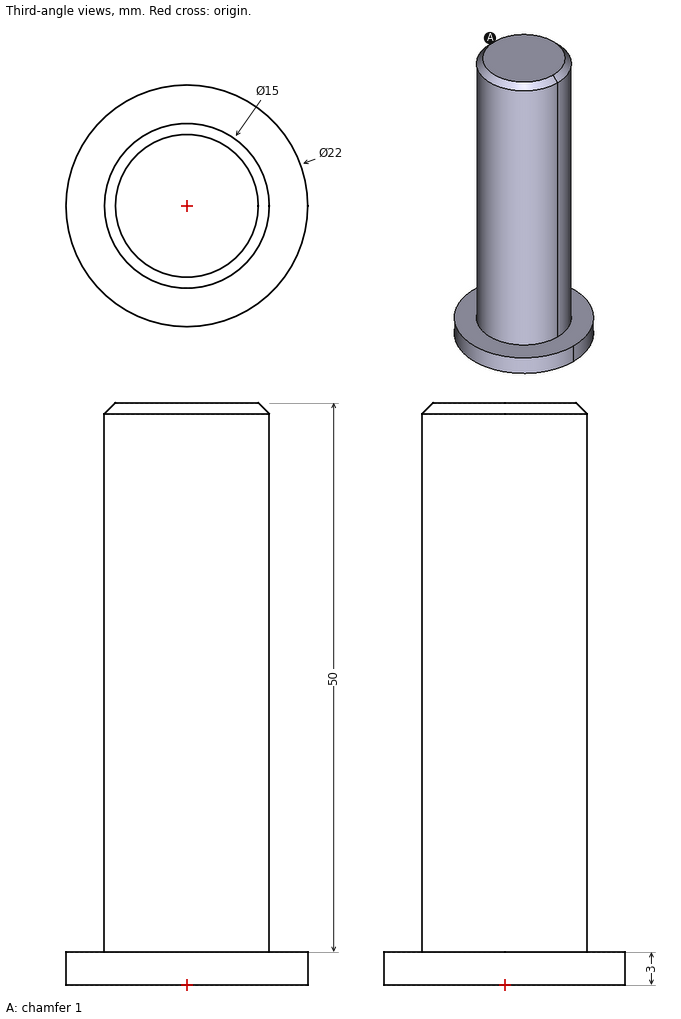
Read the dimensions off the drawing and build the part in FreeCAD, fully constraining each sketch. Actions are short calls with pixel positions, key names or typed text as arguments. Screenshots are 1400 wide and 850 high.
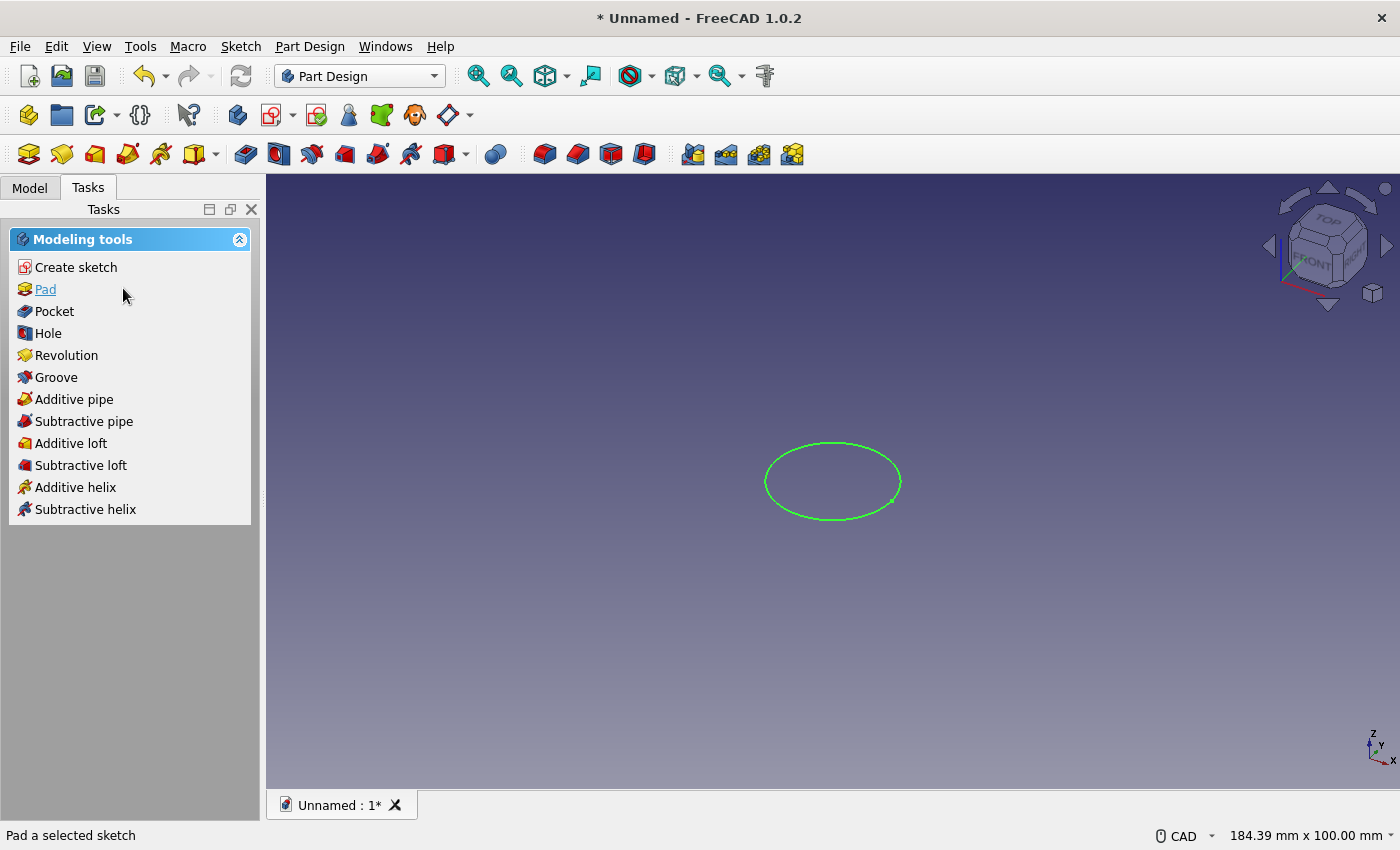
click(29, 154)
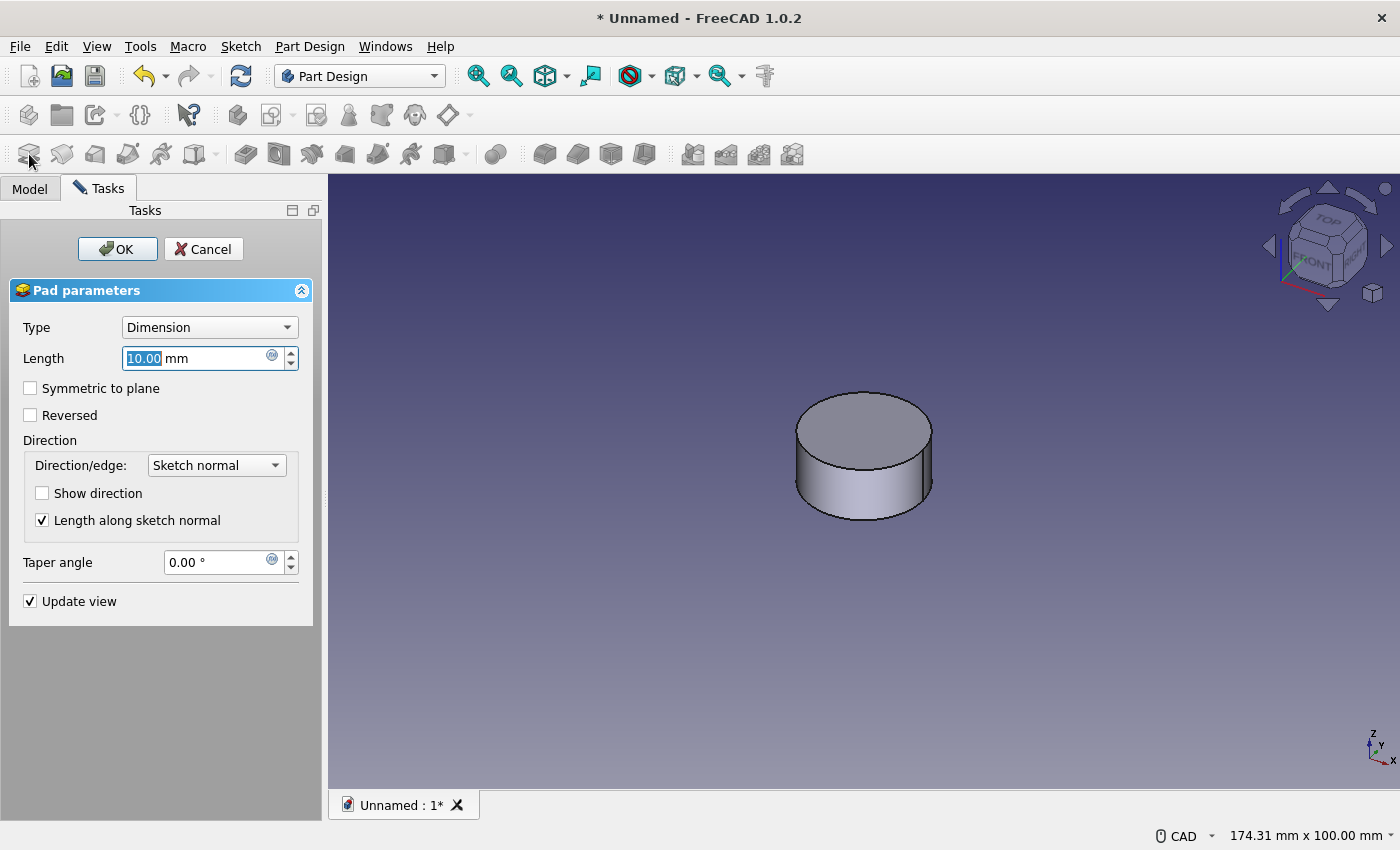
text(3)
key(Tab)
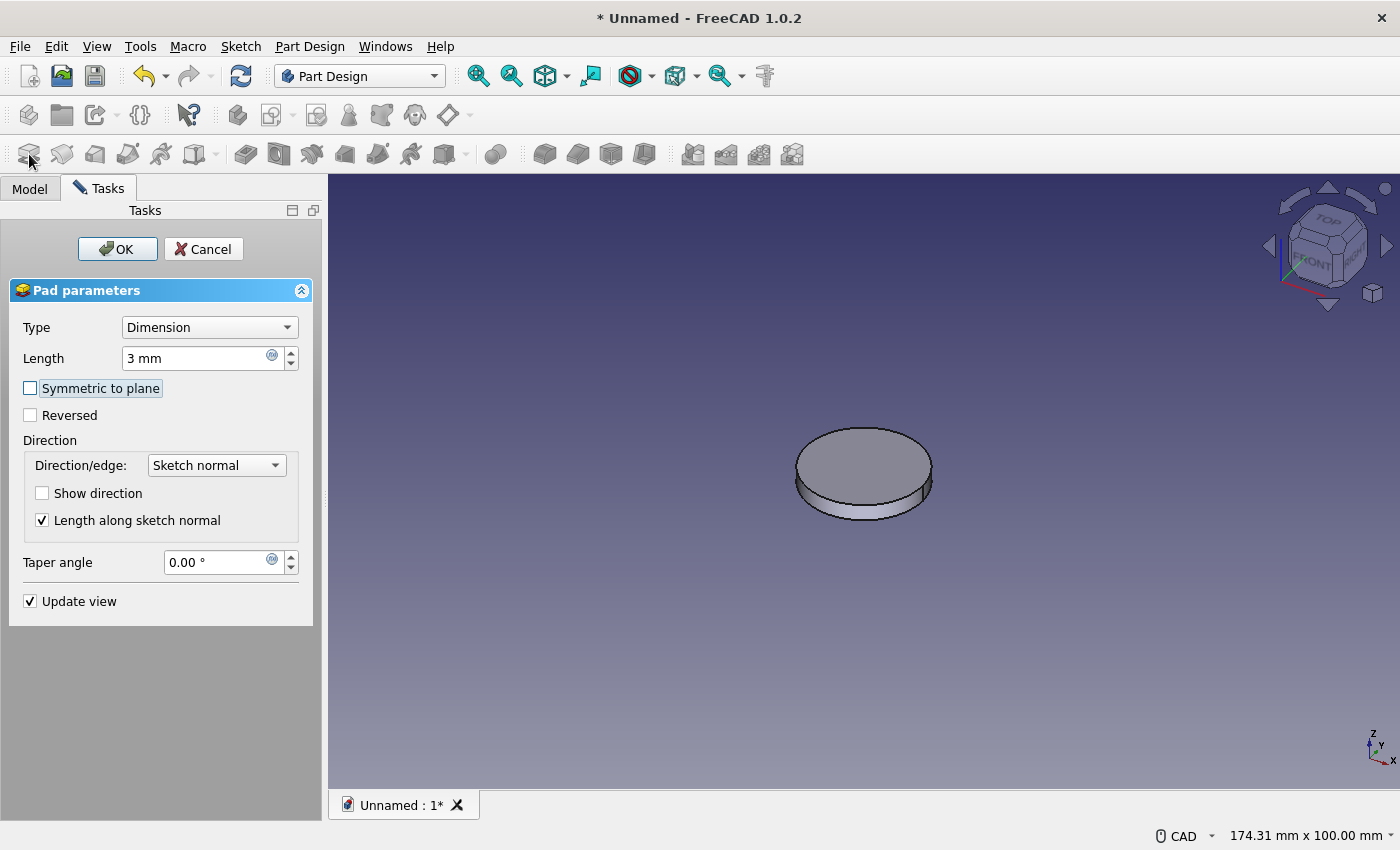
click(118, 249)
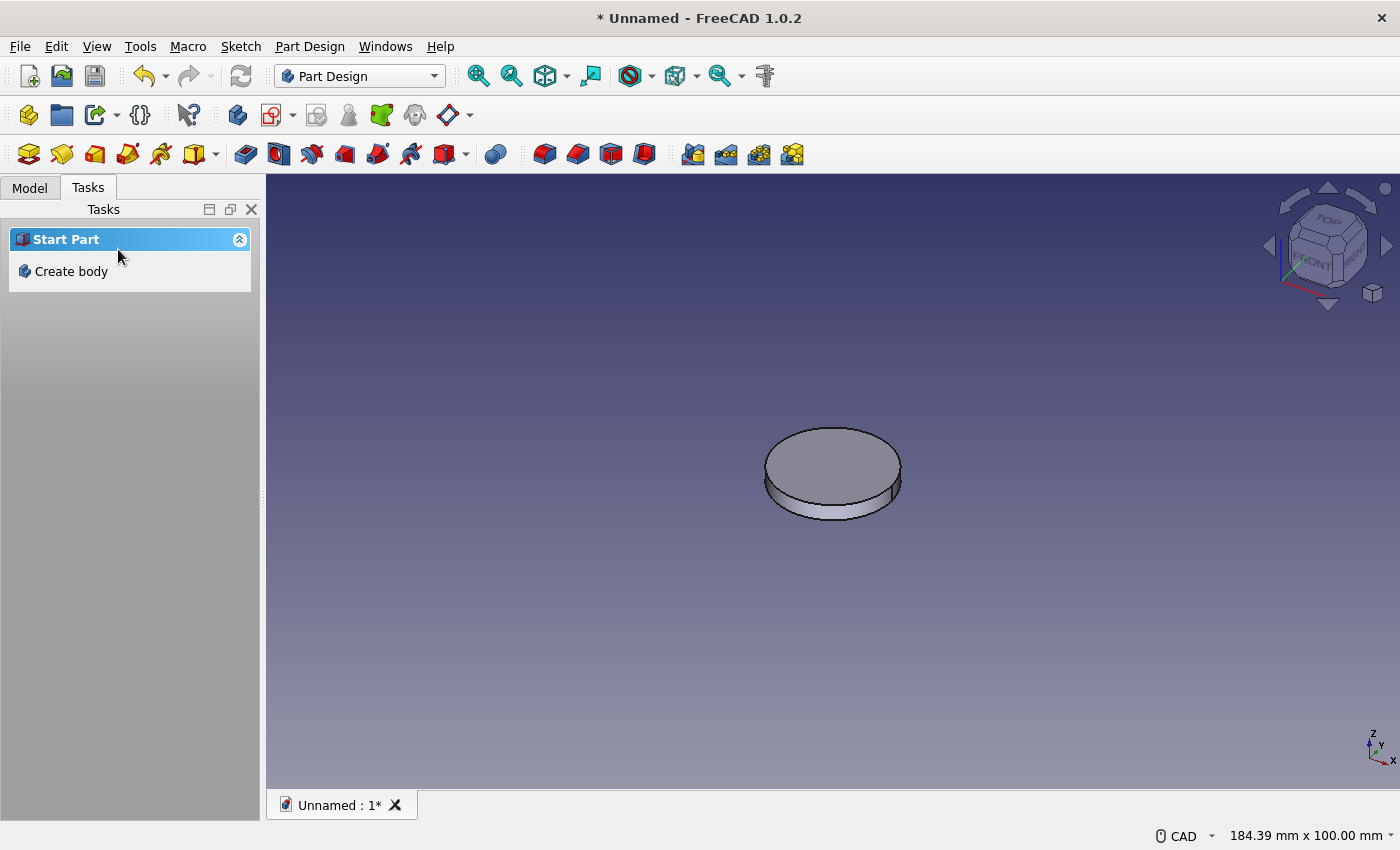
click(479, 76)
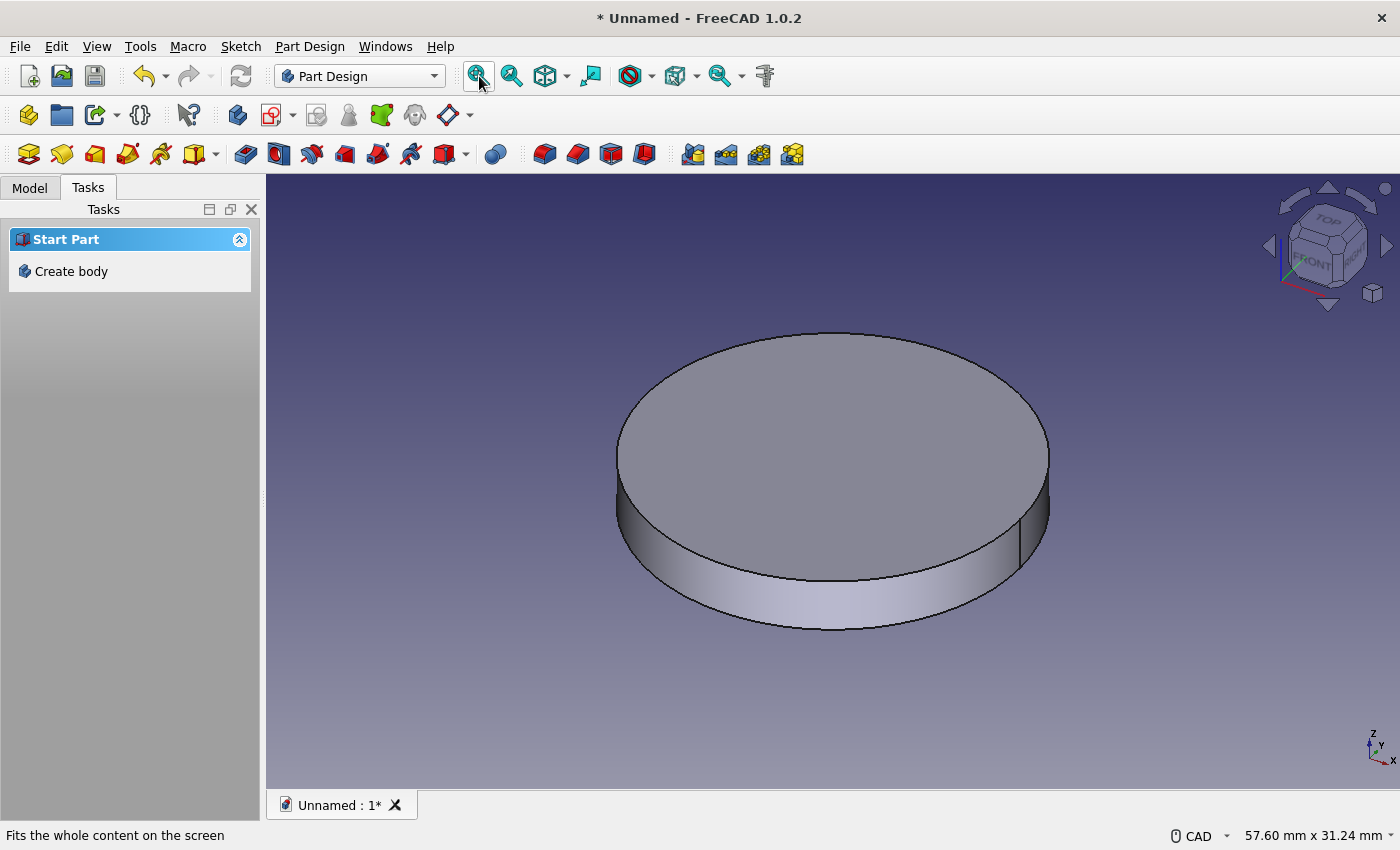
click(833, 456)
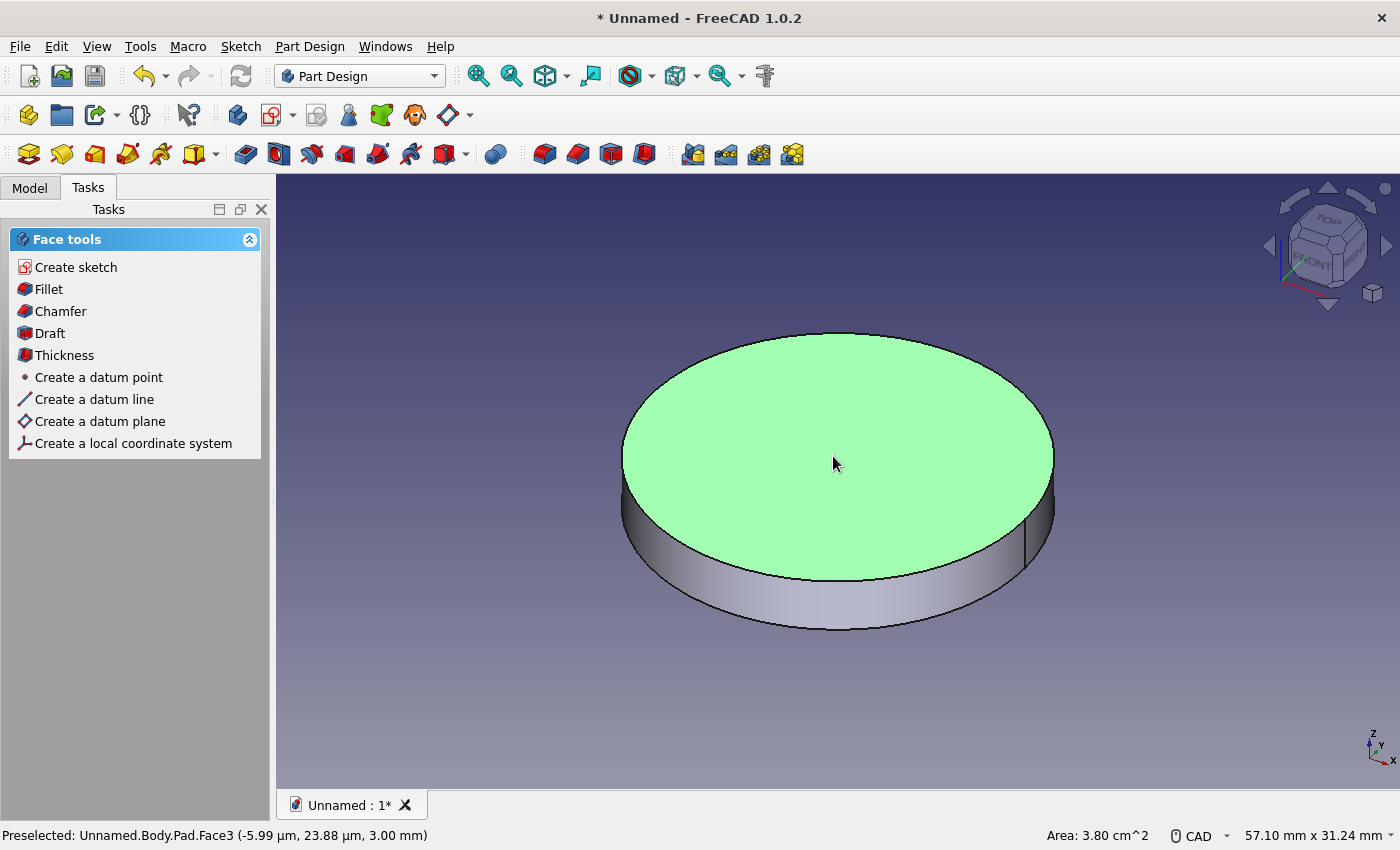
click(270, 116)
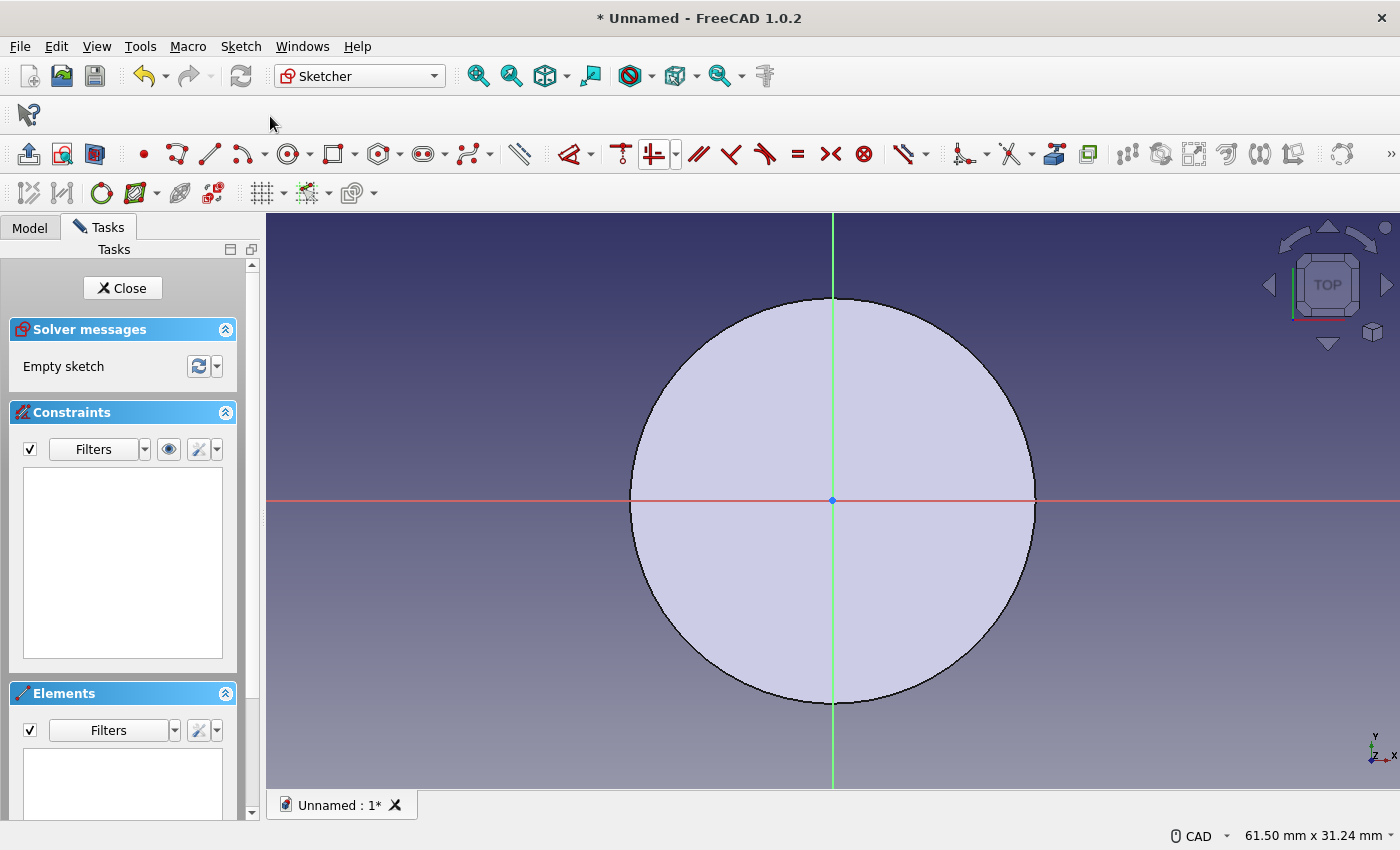
click(288, 154)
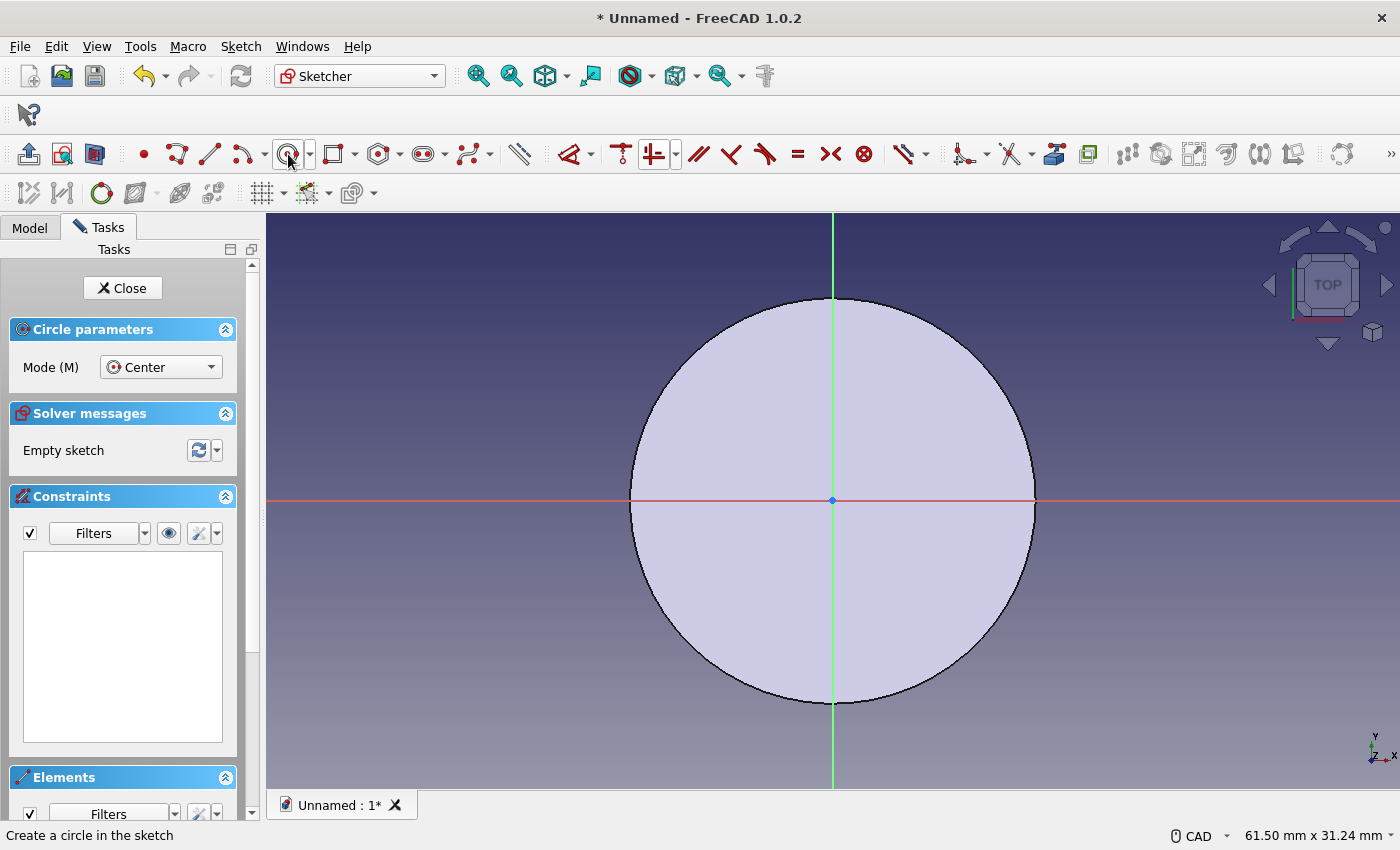
click(833, 501)
move(931, 403)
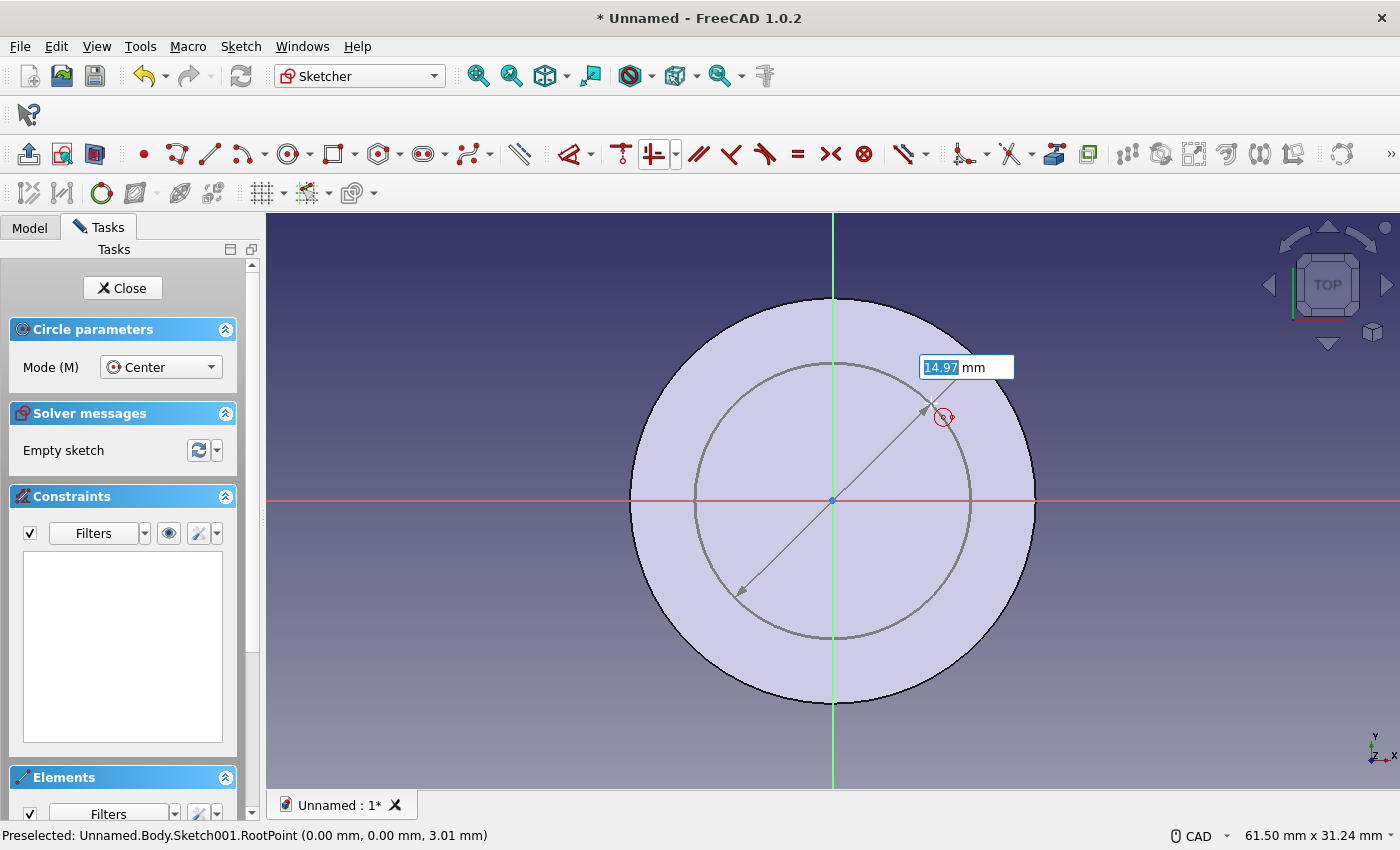
text(15)
key(Return)
key(Escape)